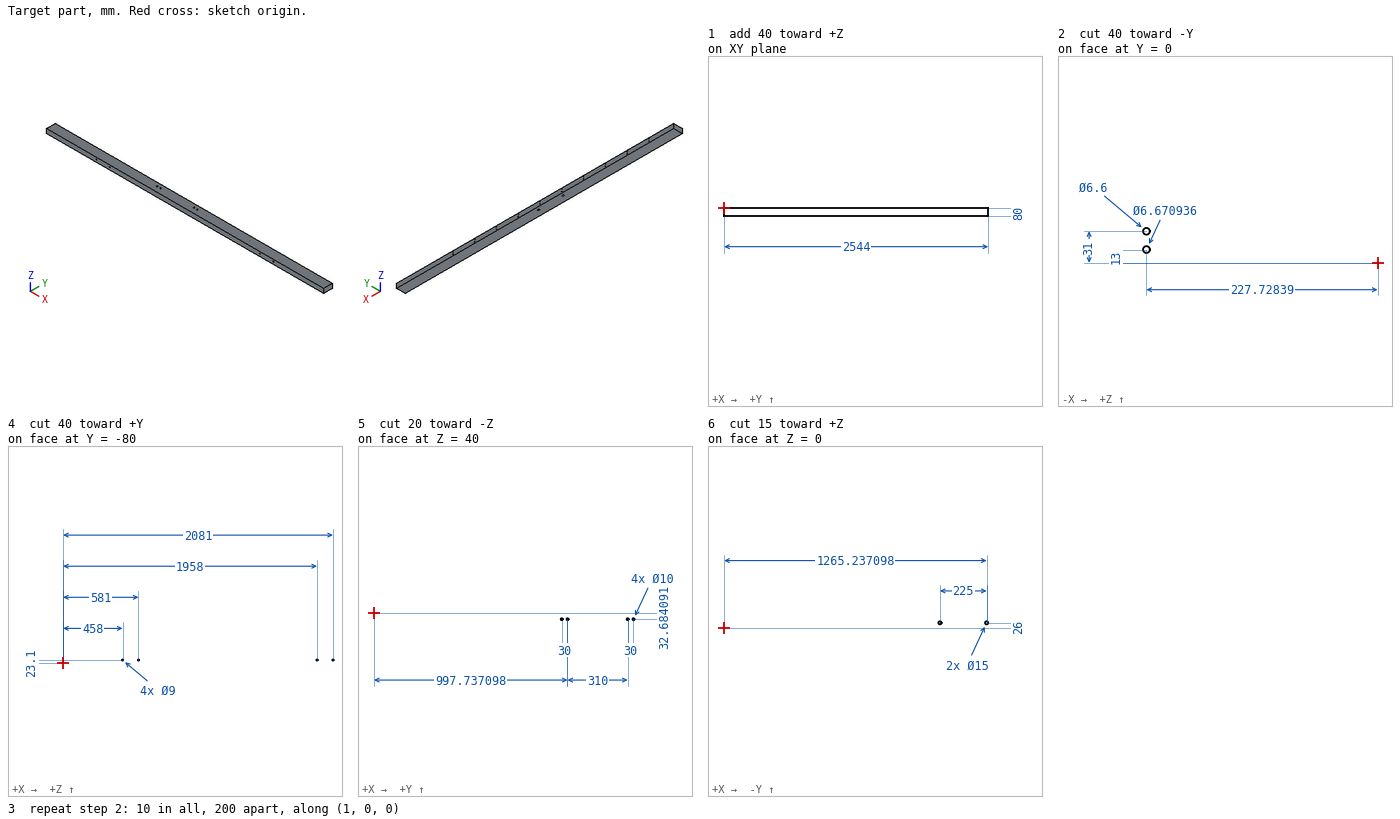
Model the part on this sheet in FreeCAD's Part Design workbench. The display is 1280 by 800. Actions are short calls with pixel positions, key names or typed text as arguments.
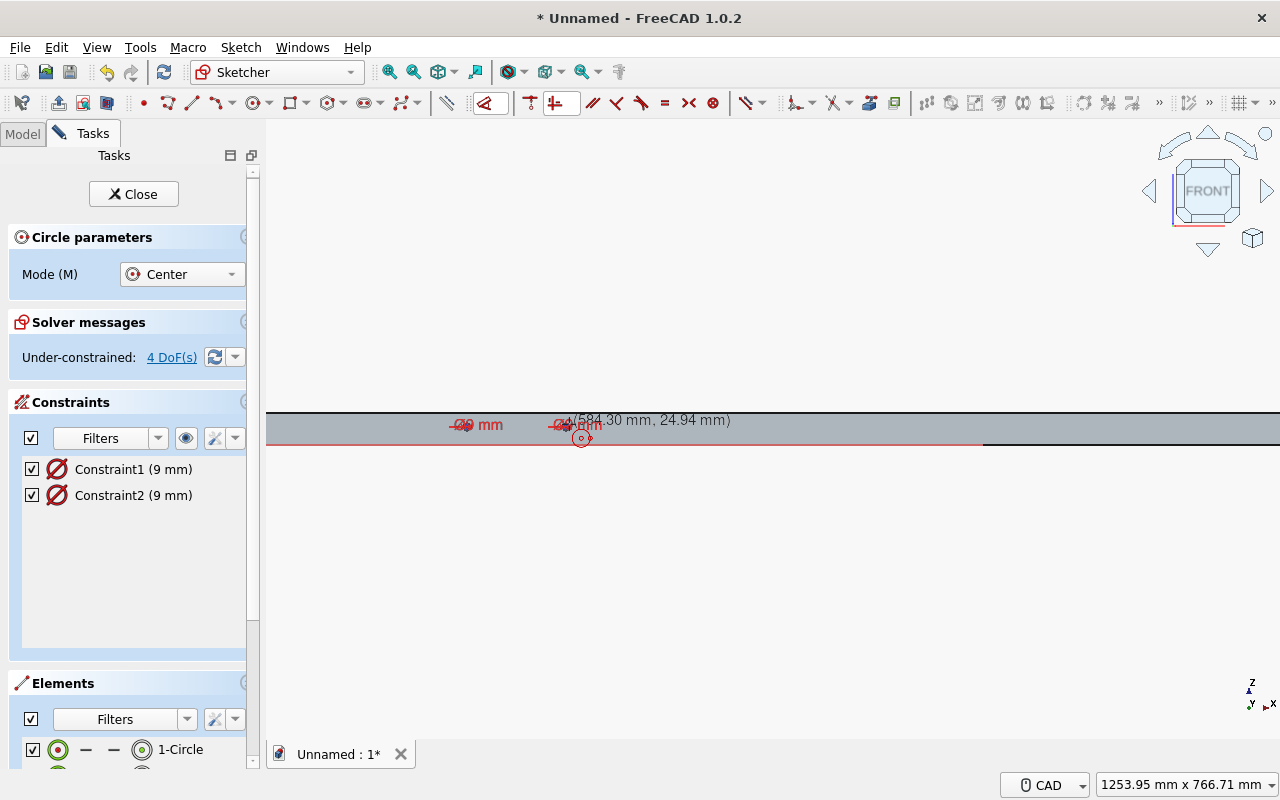
scroll(568, 426, down, 5)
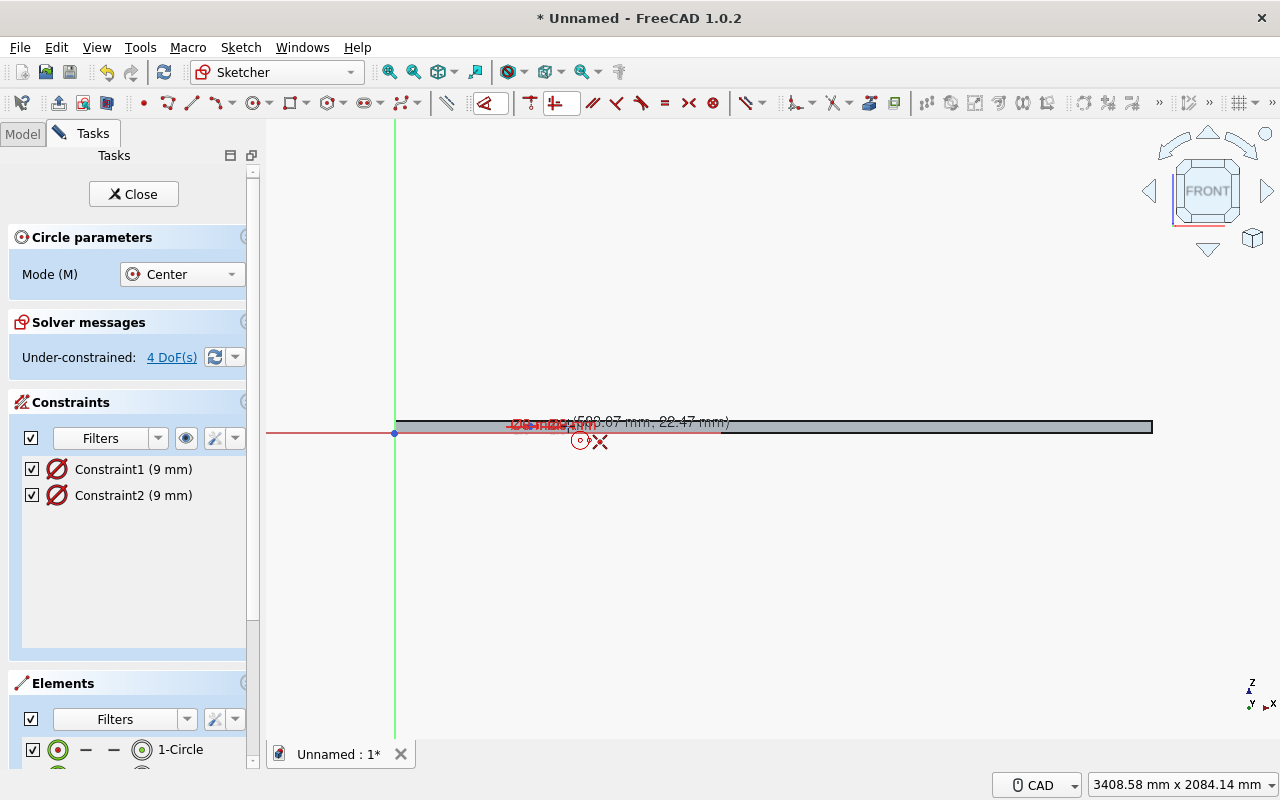
scroll(977, 426, up, 15)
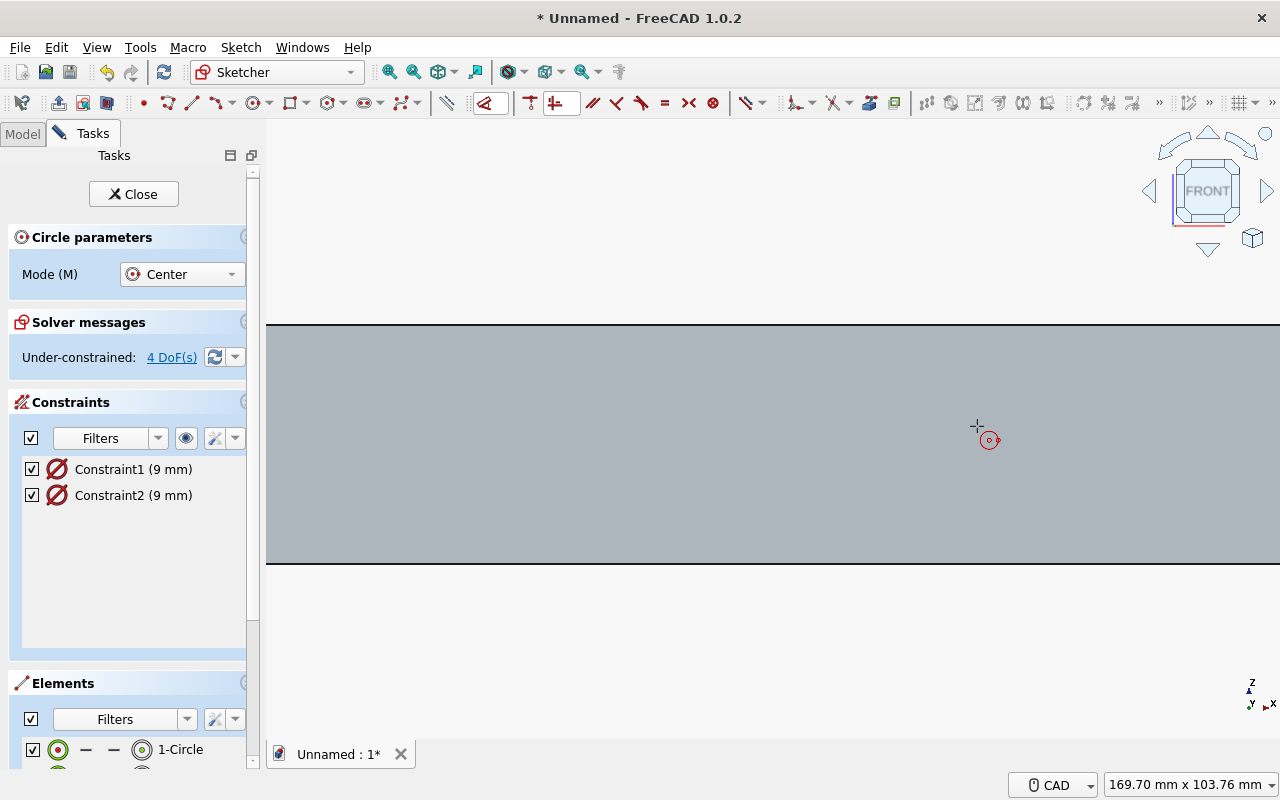
scroll(977, 426, down, 15)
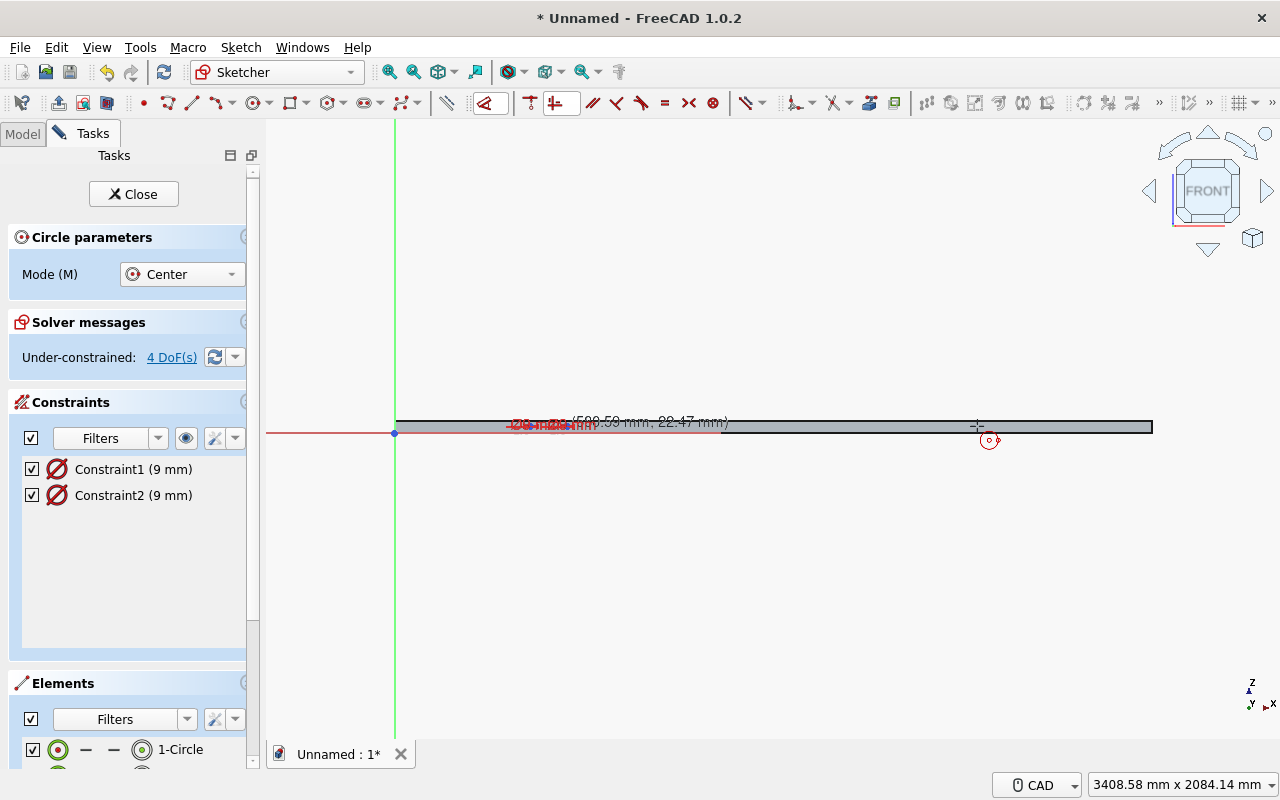
scroll(977, 426, up, 5)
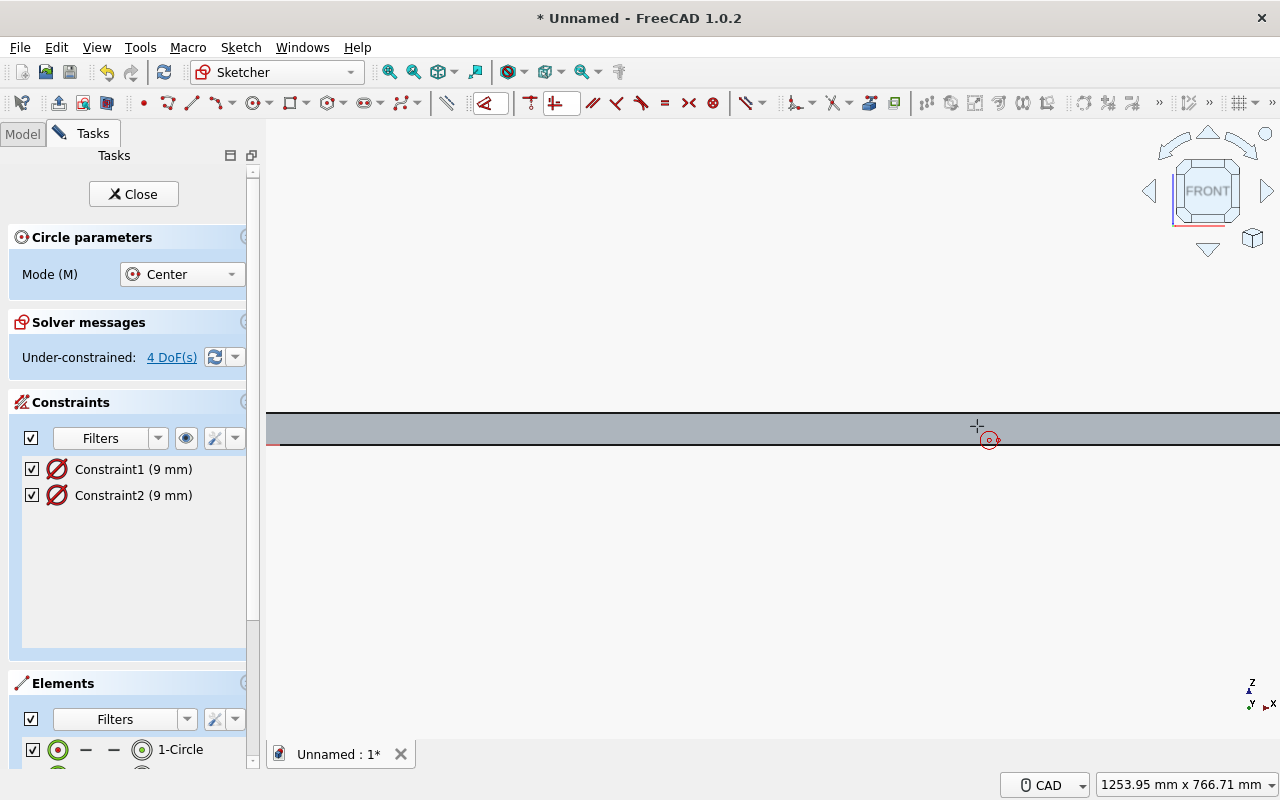
click(976, 426)
move(979, 424)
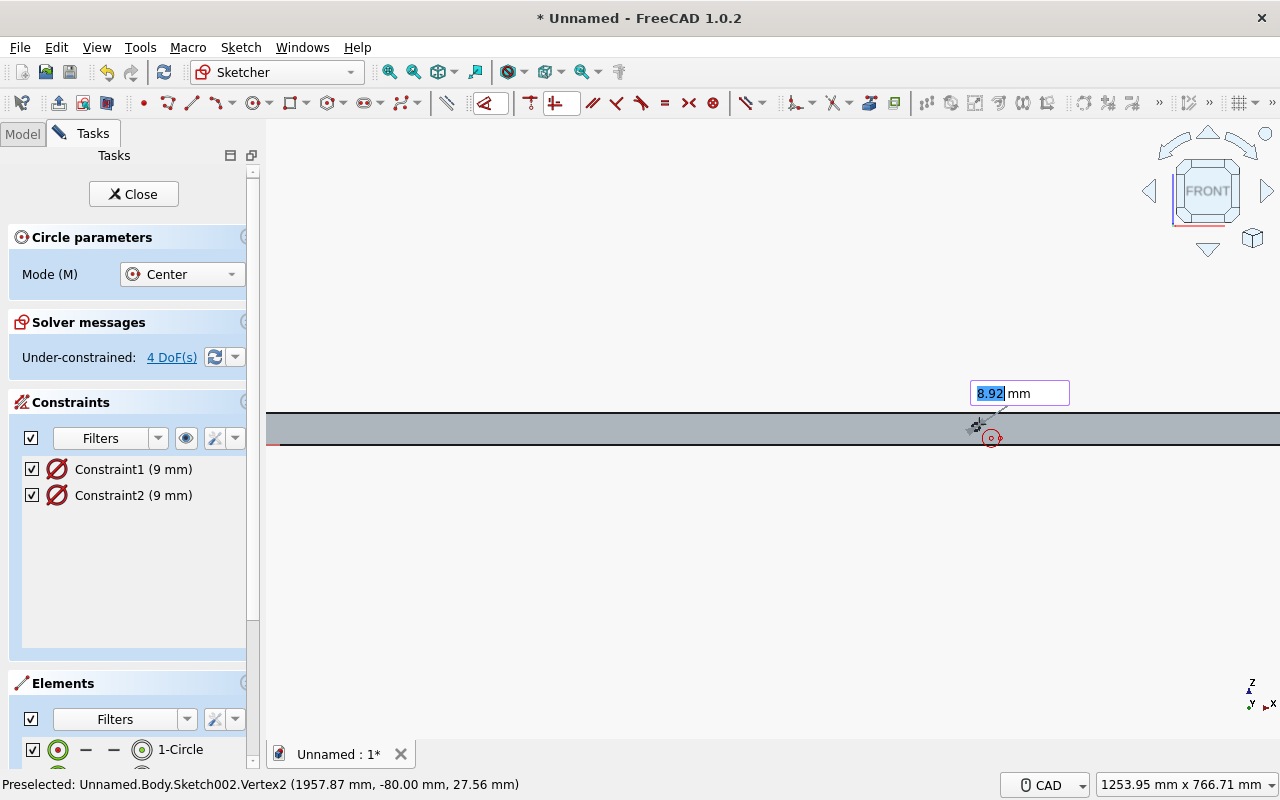
text(9)
key(Return)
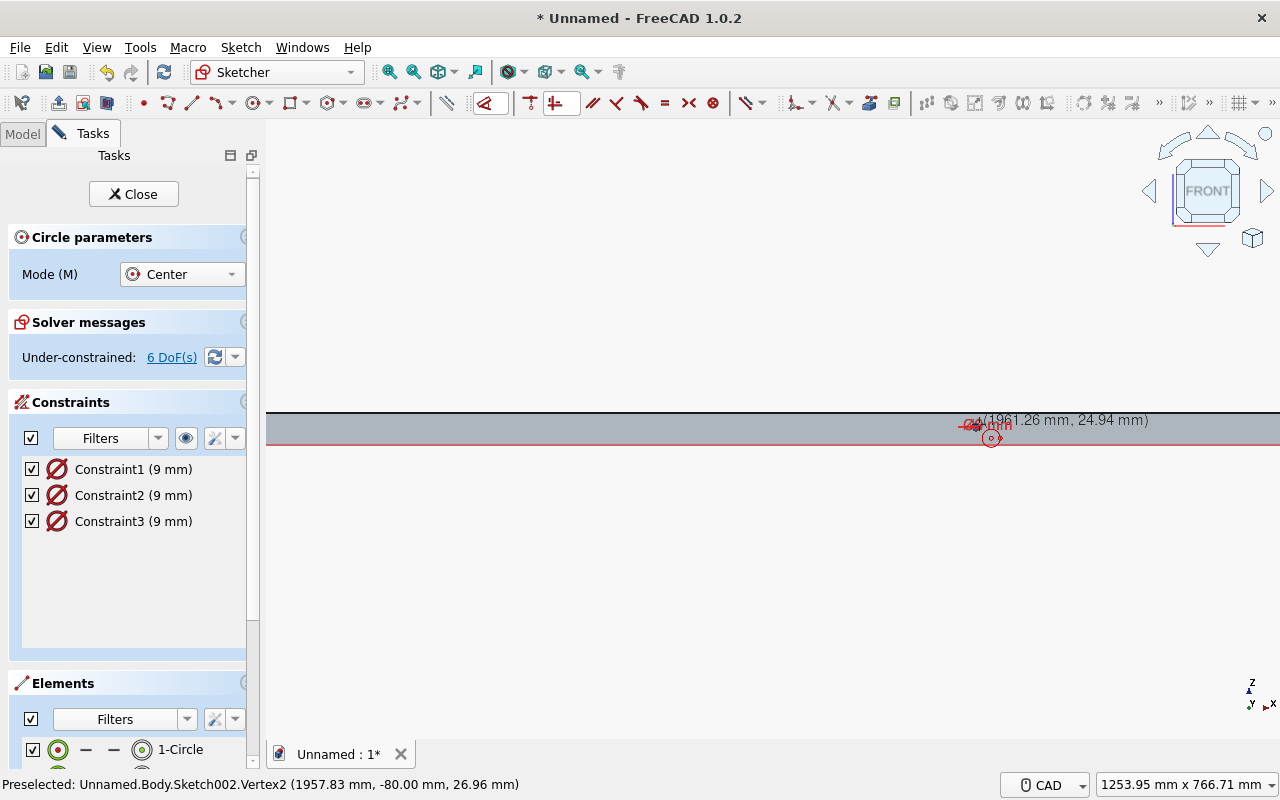
scroll(1076, 426, up, 10)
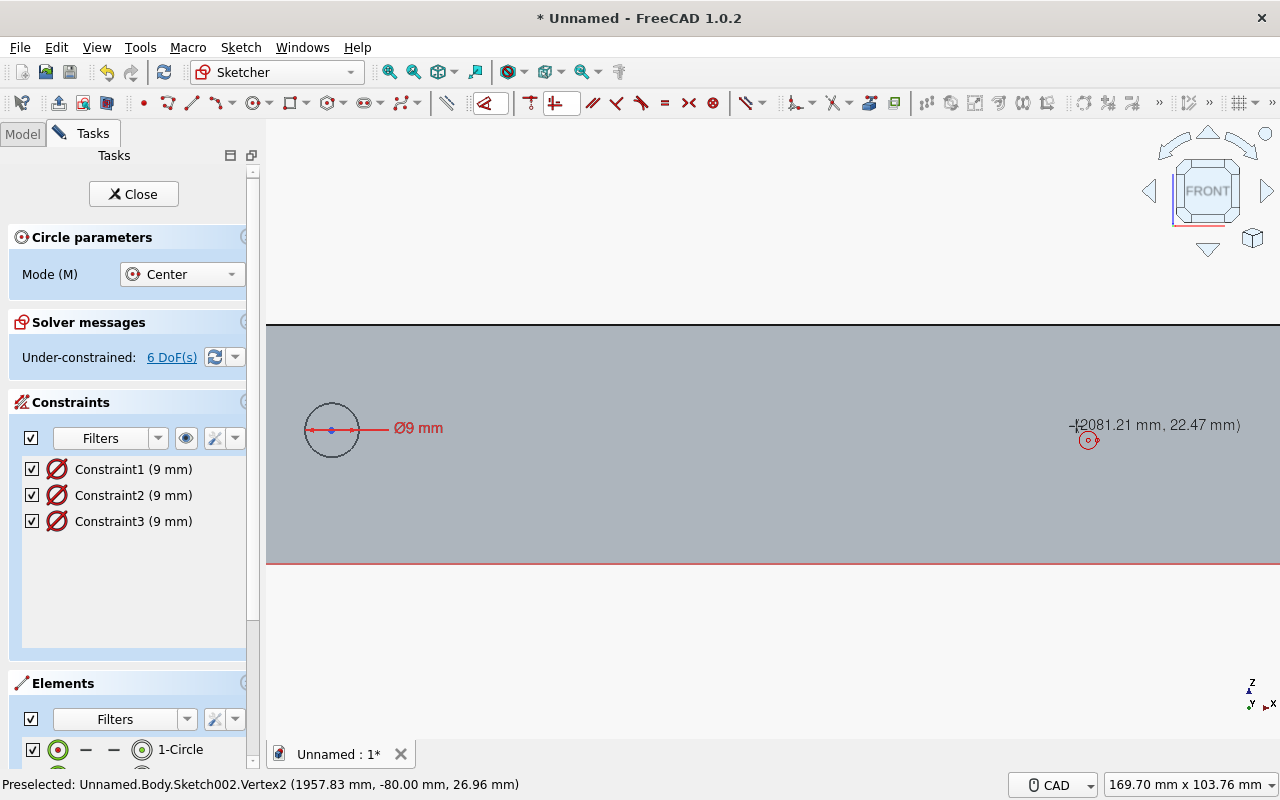
scroll(1010, 426, down, 15)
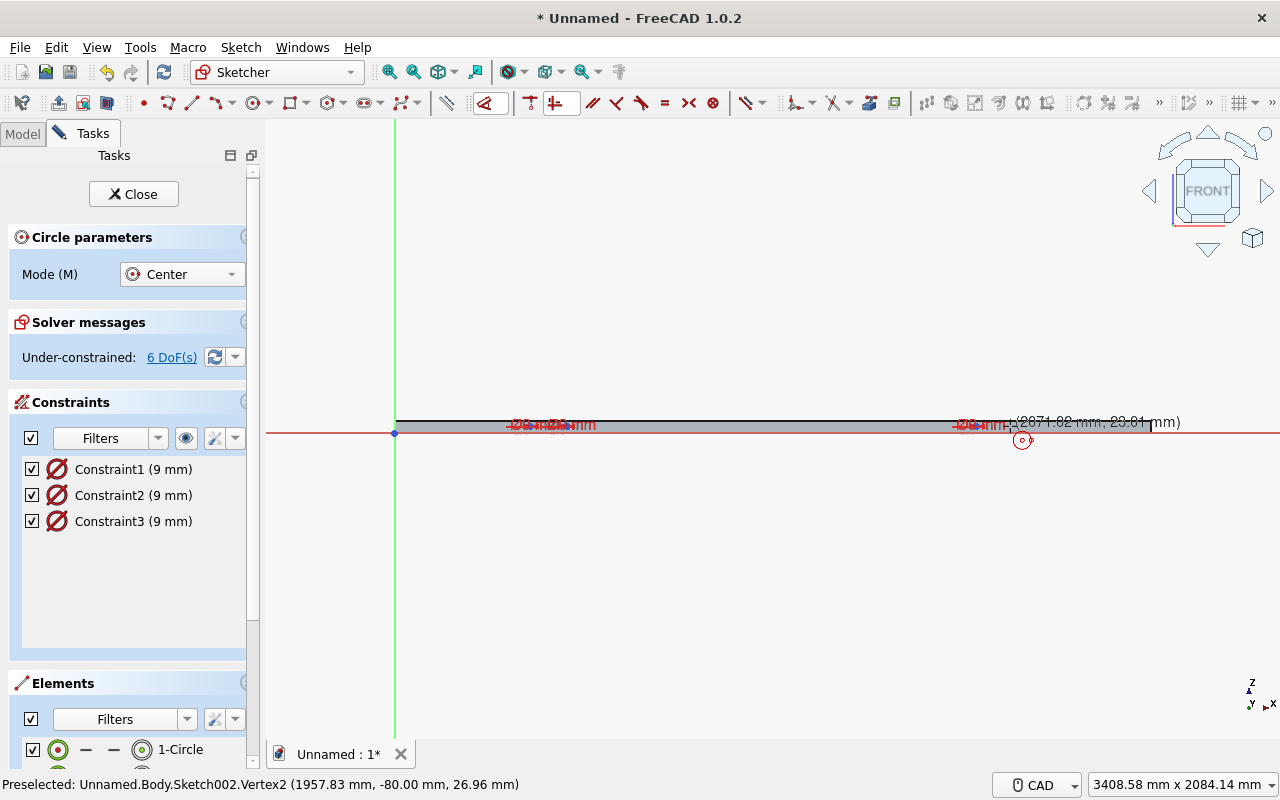
scroll(1014, 426, up, 5)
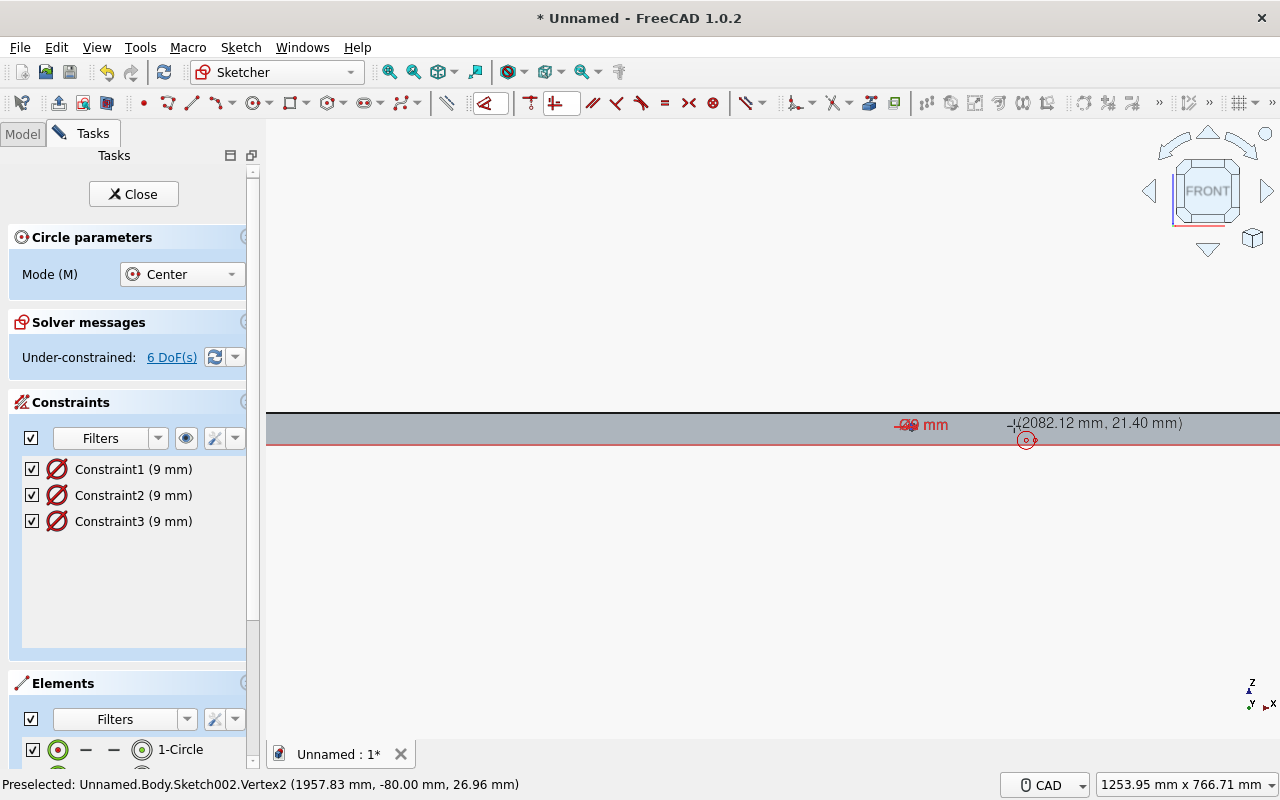
click(1012, 426)
move(1014, 424)